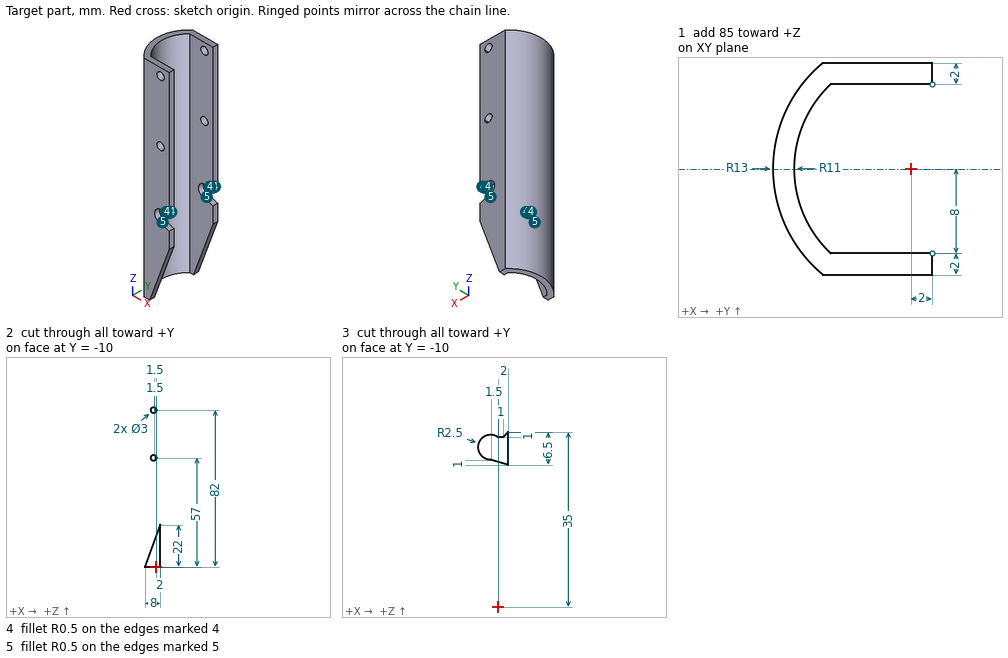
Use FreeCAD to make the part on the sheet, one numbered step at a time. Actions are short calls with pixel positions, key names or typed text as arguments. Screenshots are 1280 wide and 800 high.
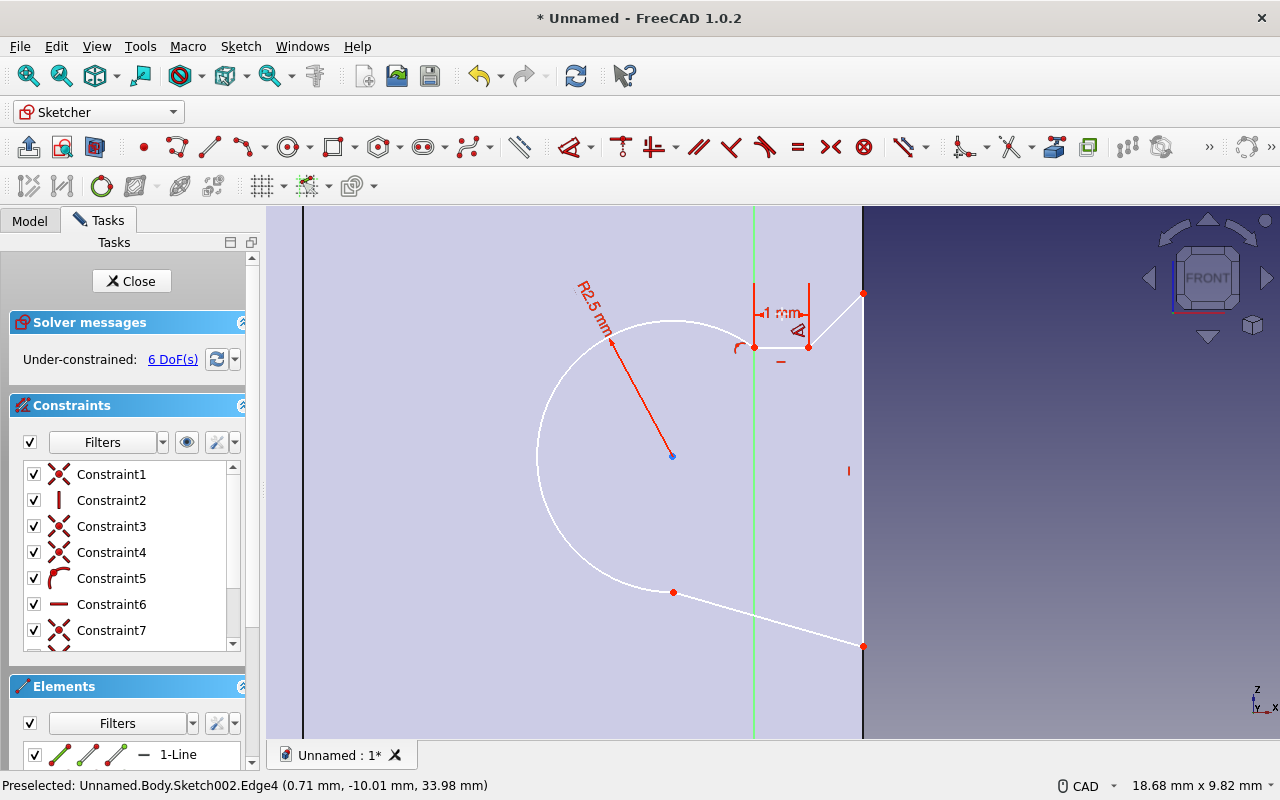
click(863, 647)
click(809, 613)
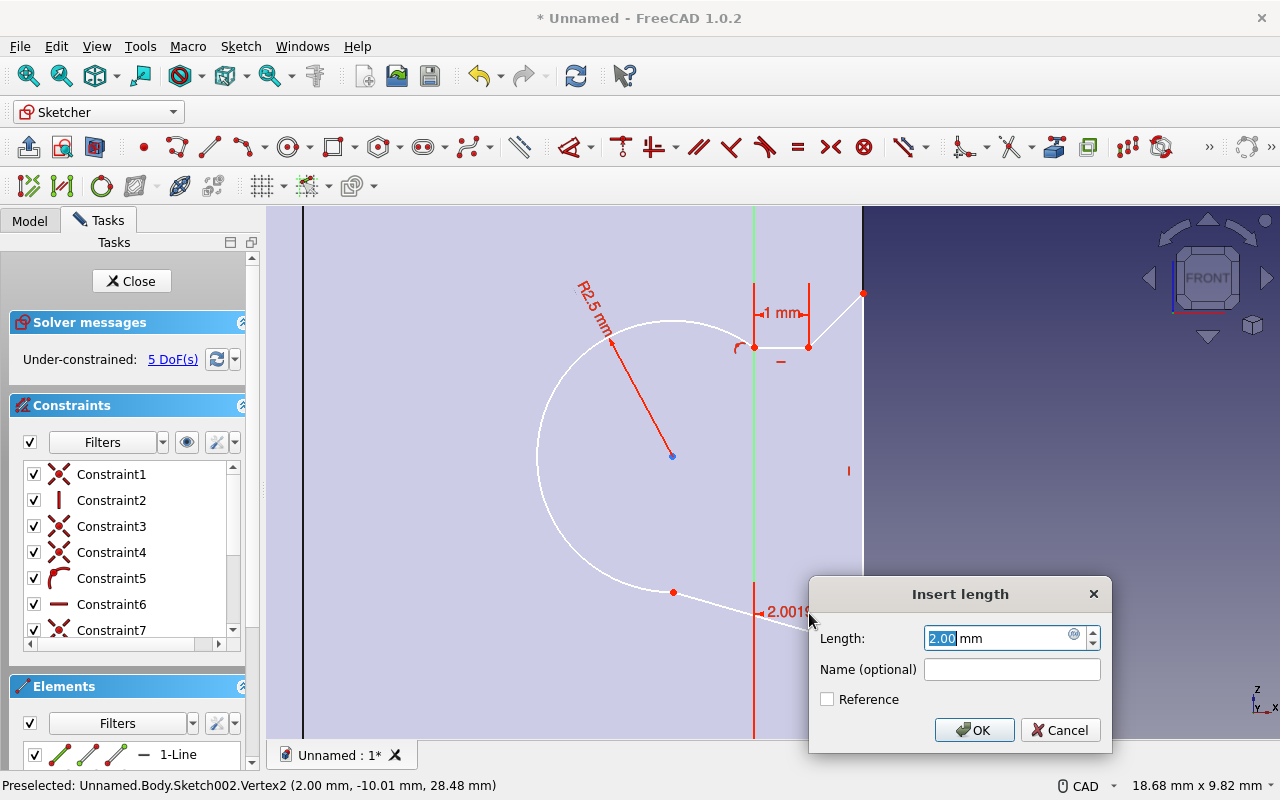
text(2)
key(Return)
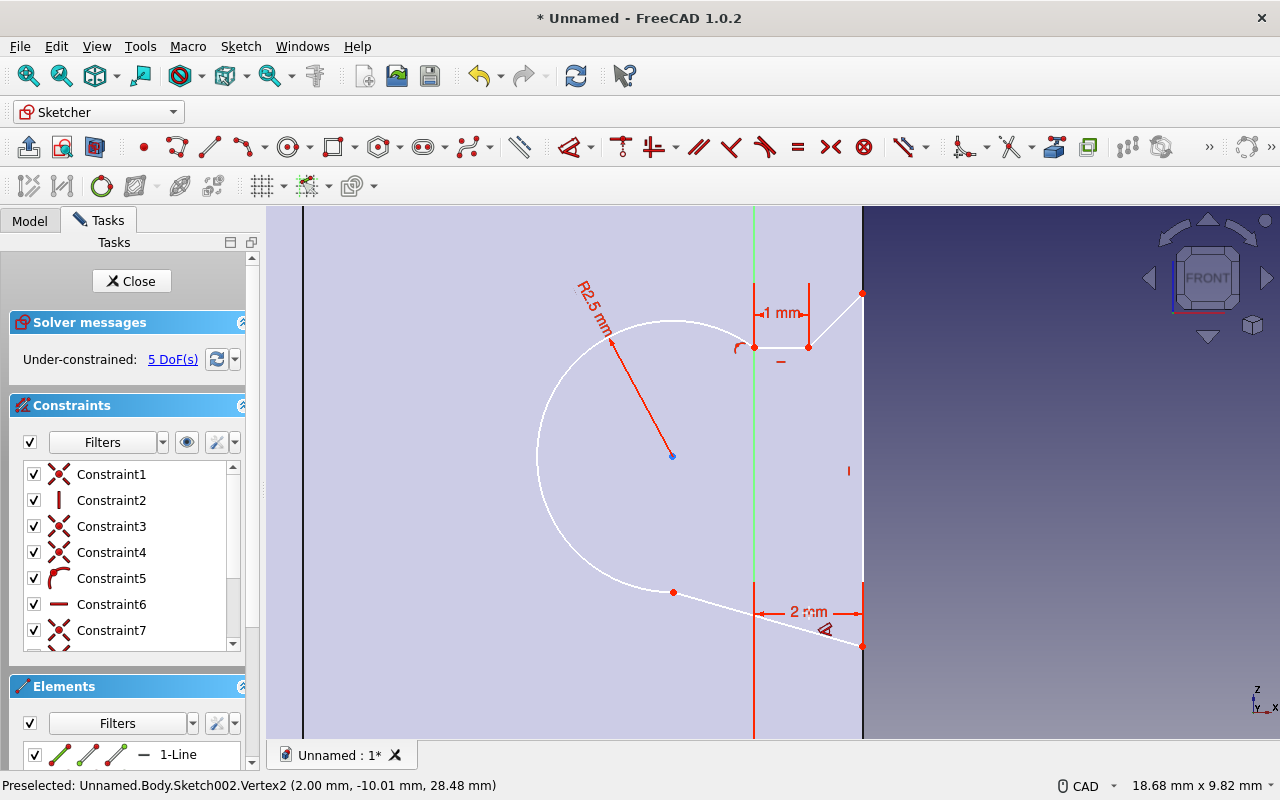
click(730, 609)
click(897, 620)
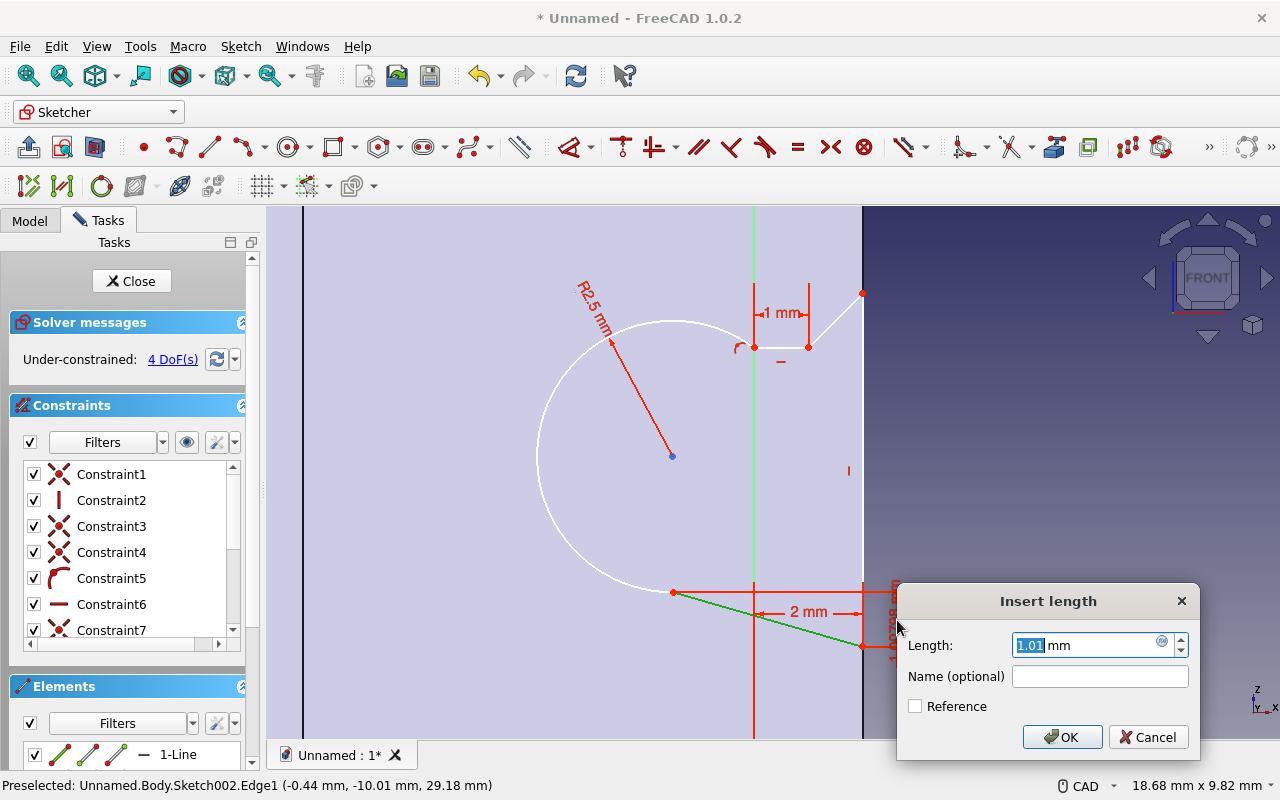
text(1)
key(Return)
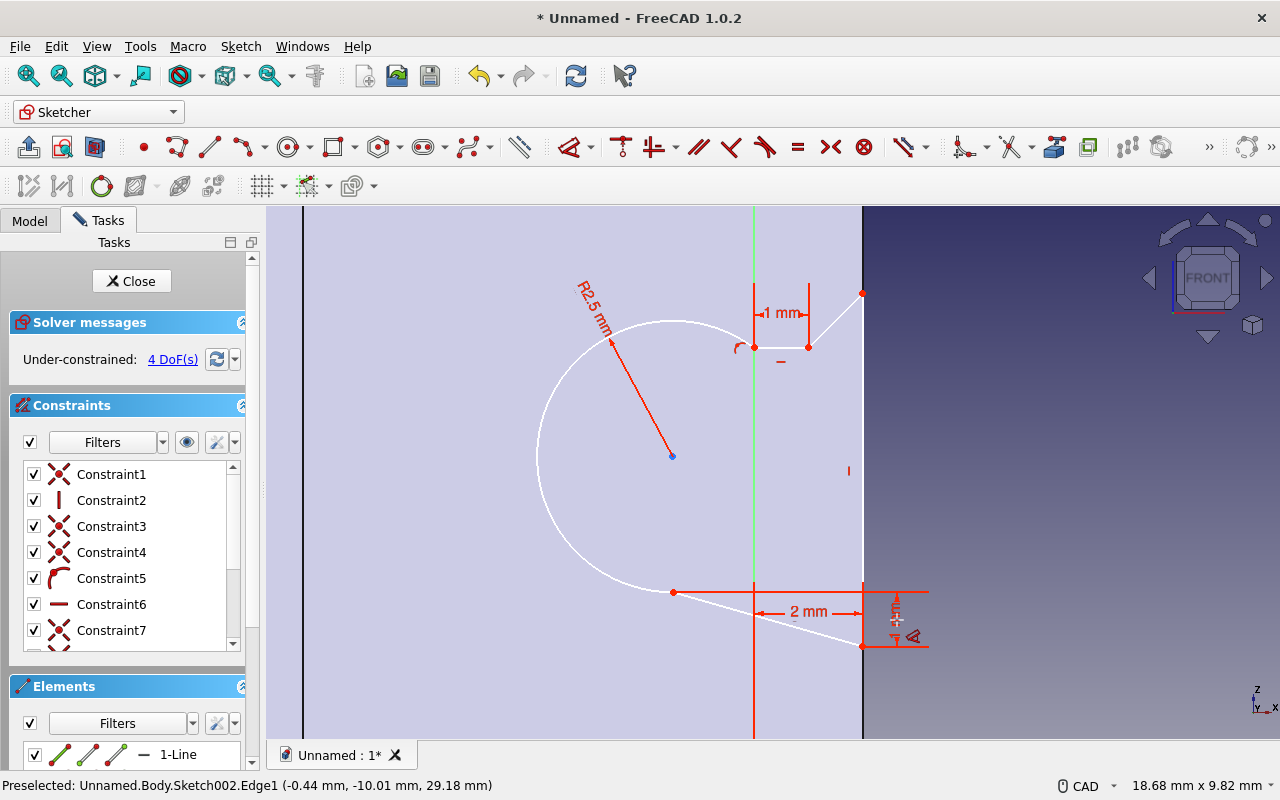
click(847, 310)
click(897, 321)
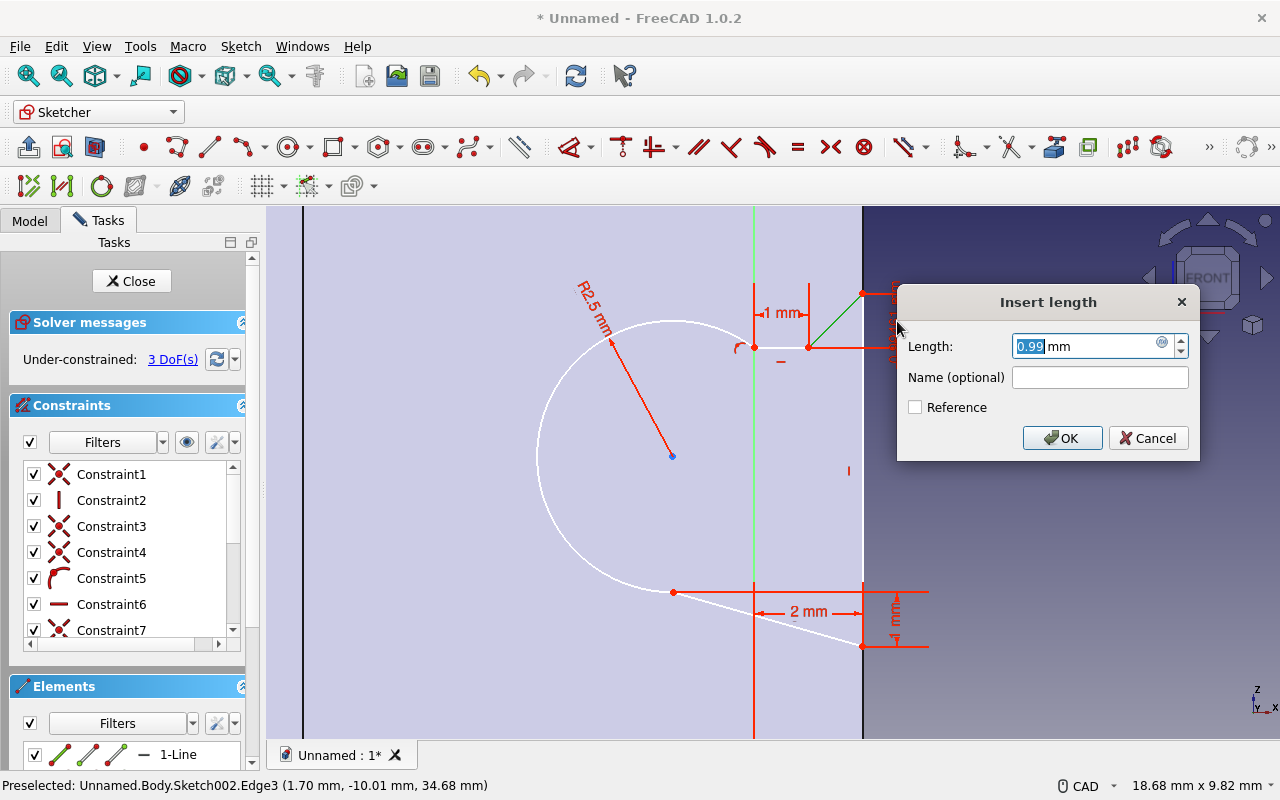
text(1)
key(Return)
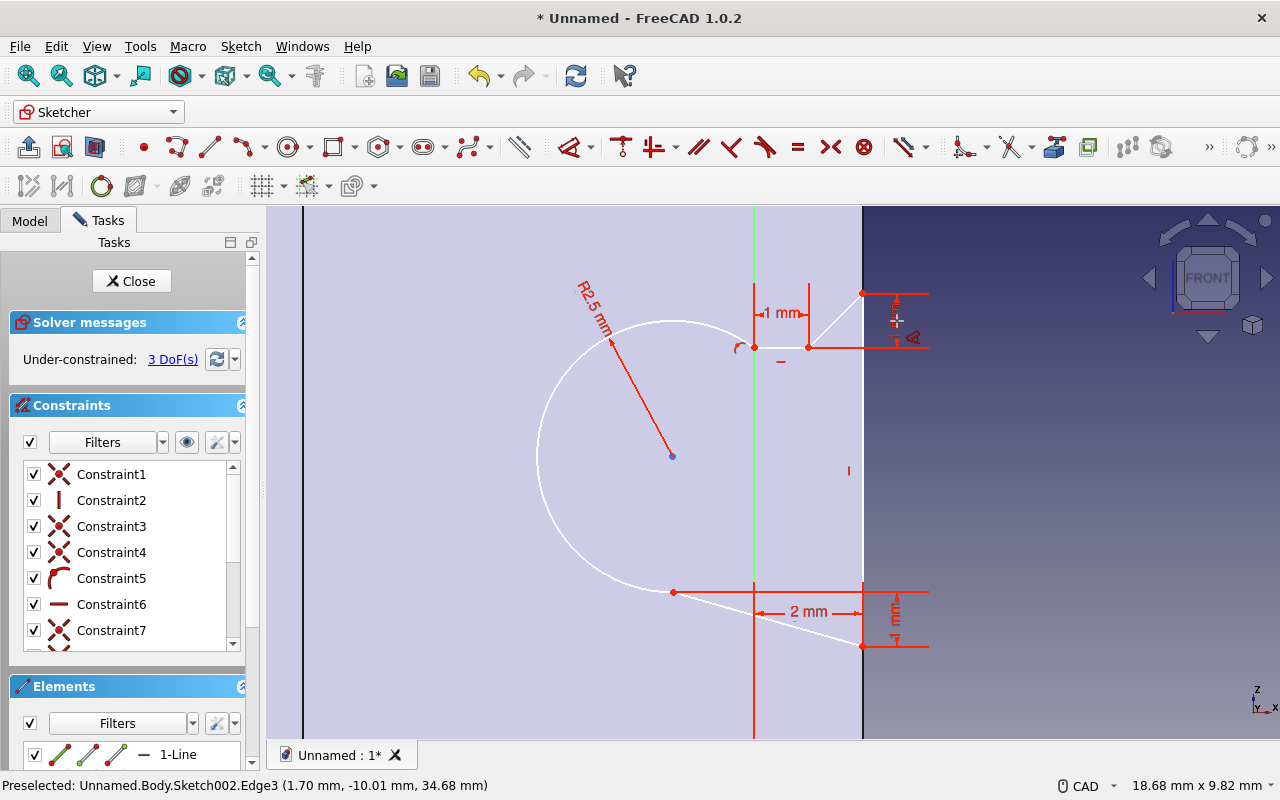
click(863, 541)
click(897, 470)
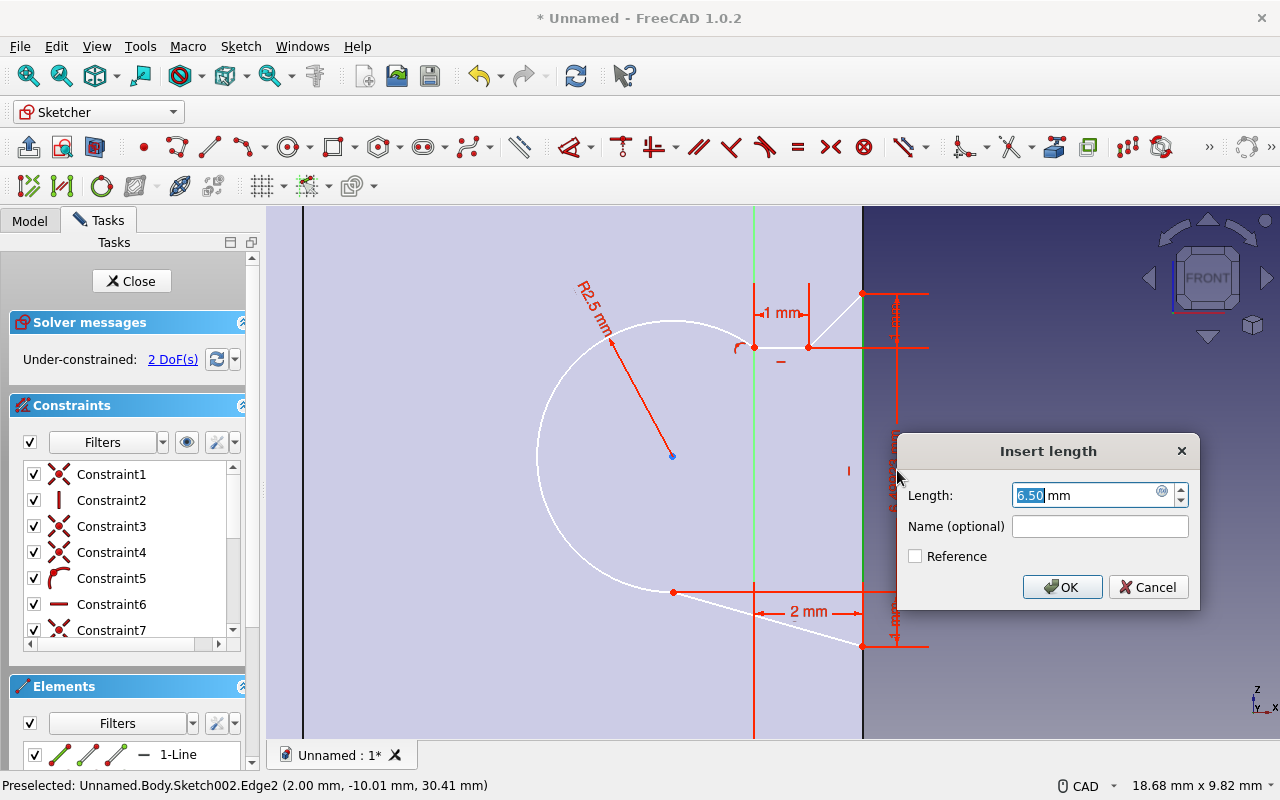
text(6.5)
key(Return)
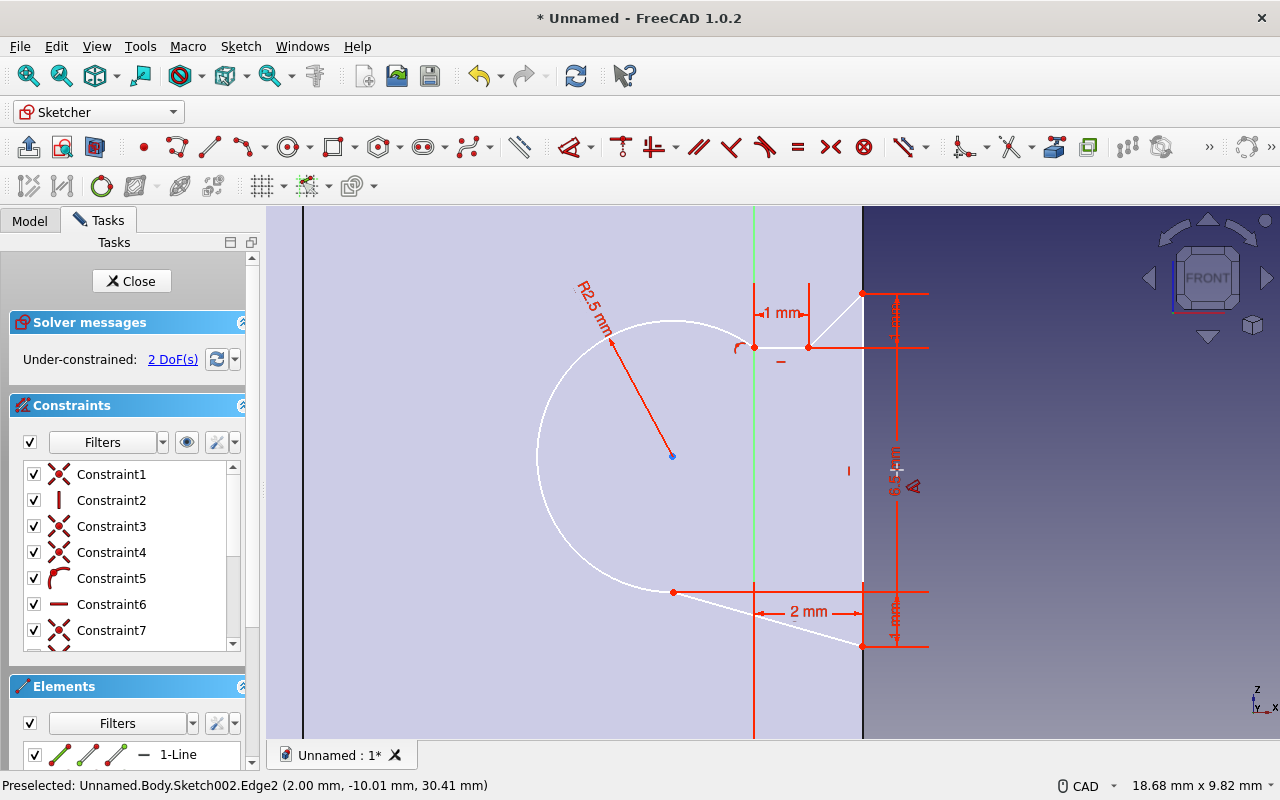
click(863, 294)
click(897, 502)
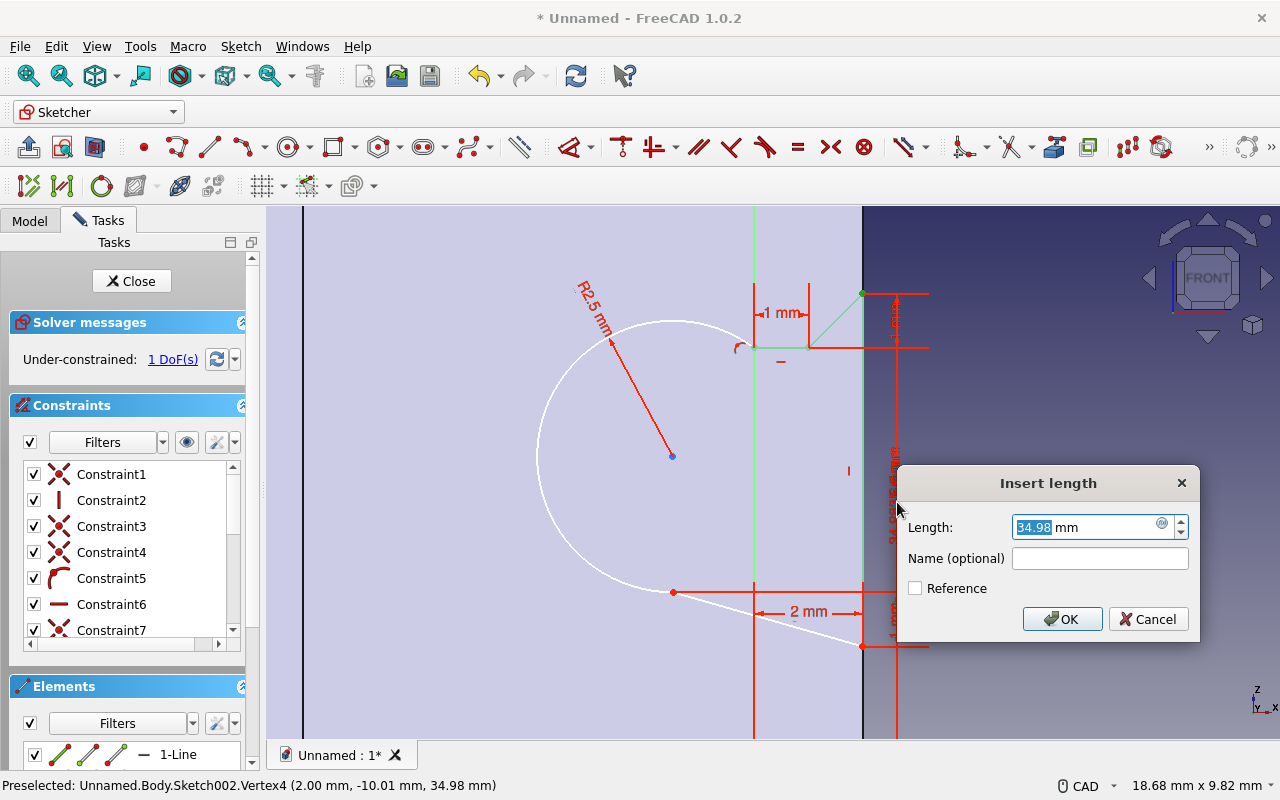
text(35)
key(Return)